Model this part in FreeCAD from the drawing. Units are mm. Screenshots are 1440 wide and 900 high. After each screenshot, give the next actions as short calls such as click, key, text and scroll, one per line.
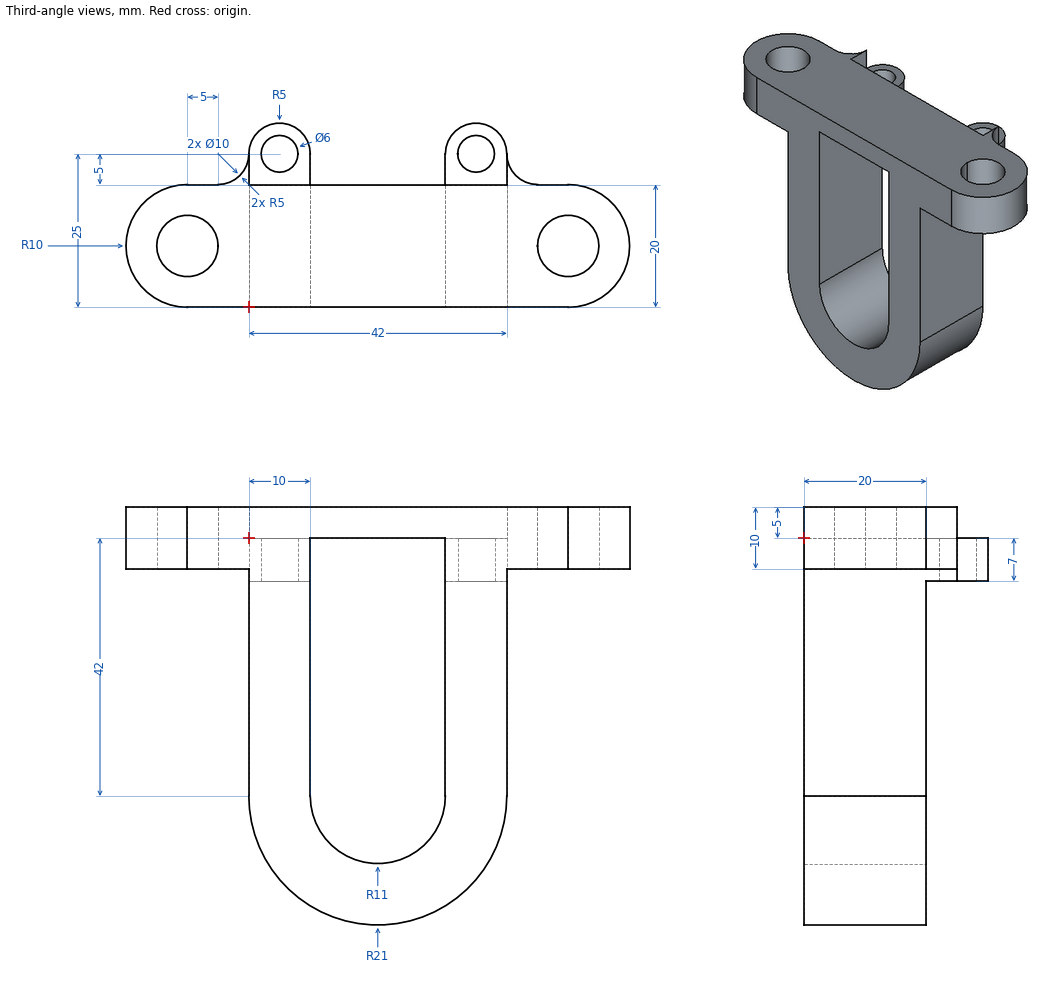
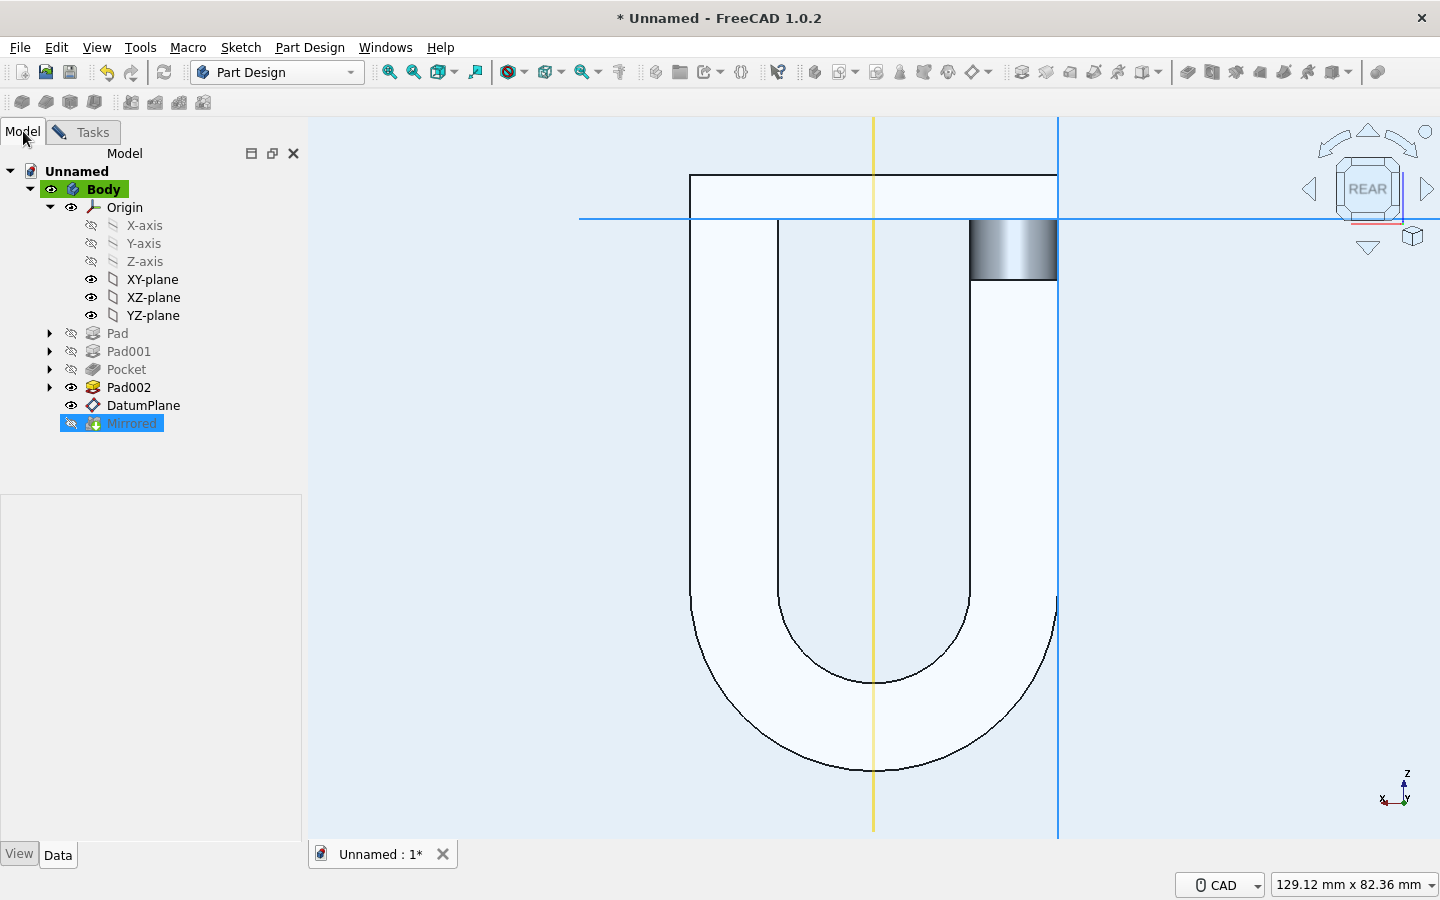
click(116, 405)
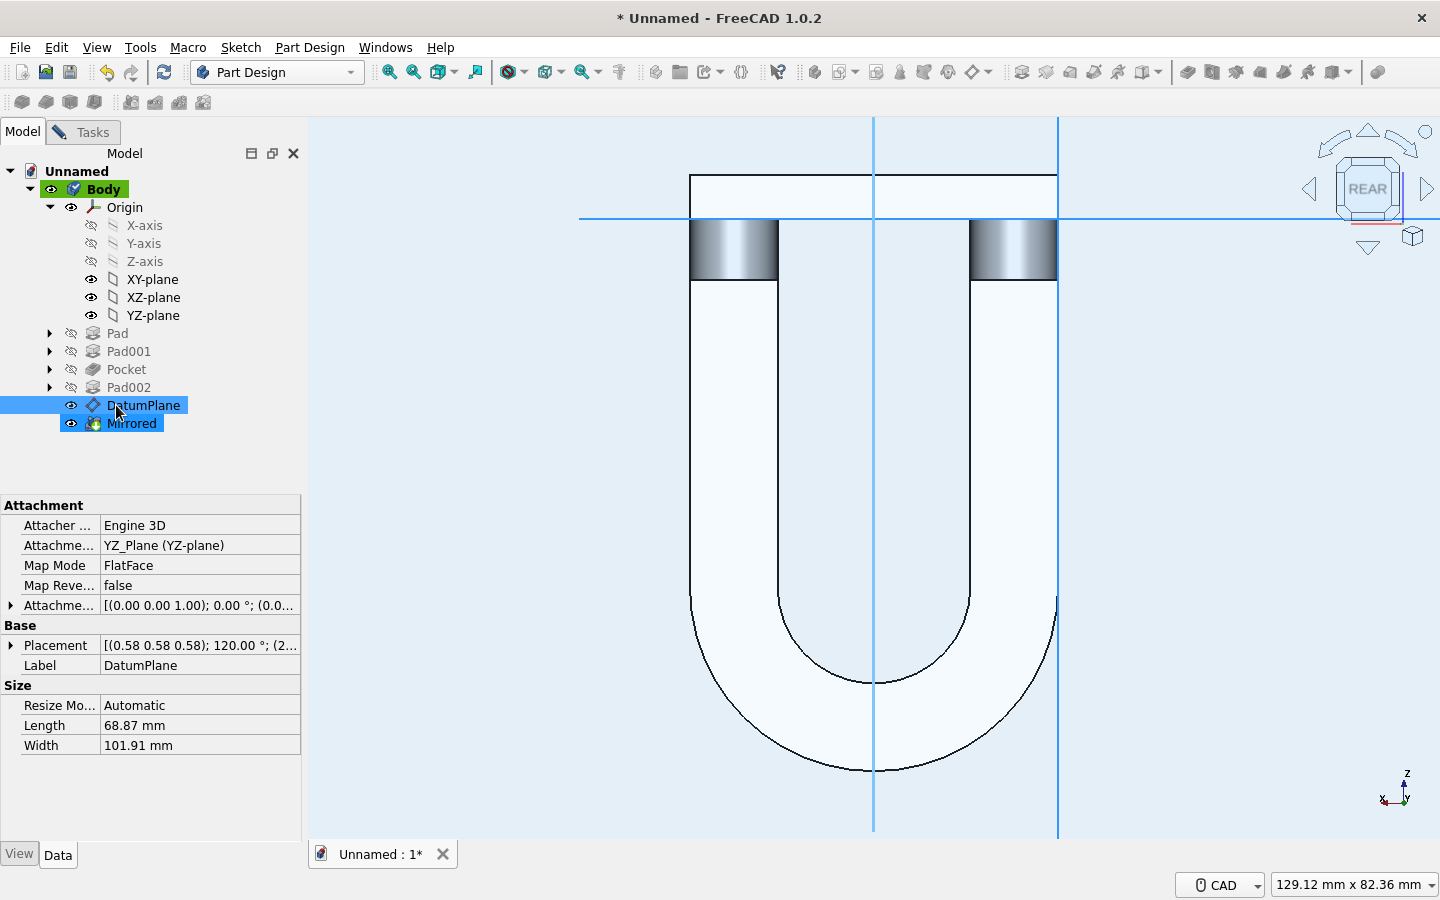
click(84, 131)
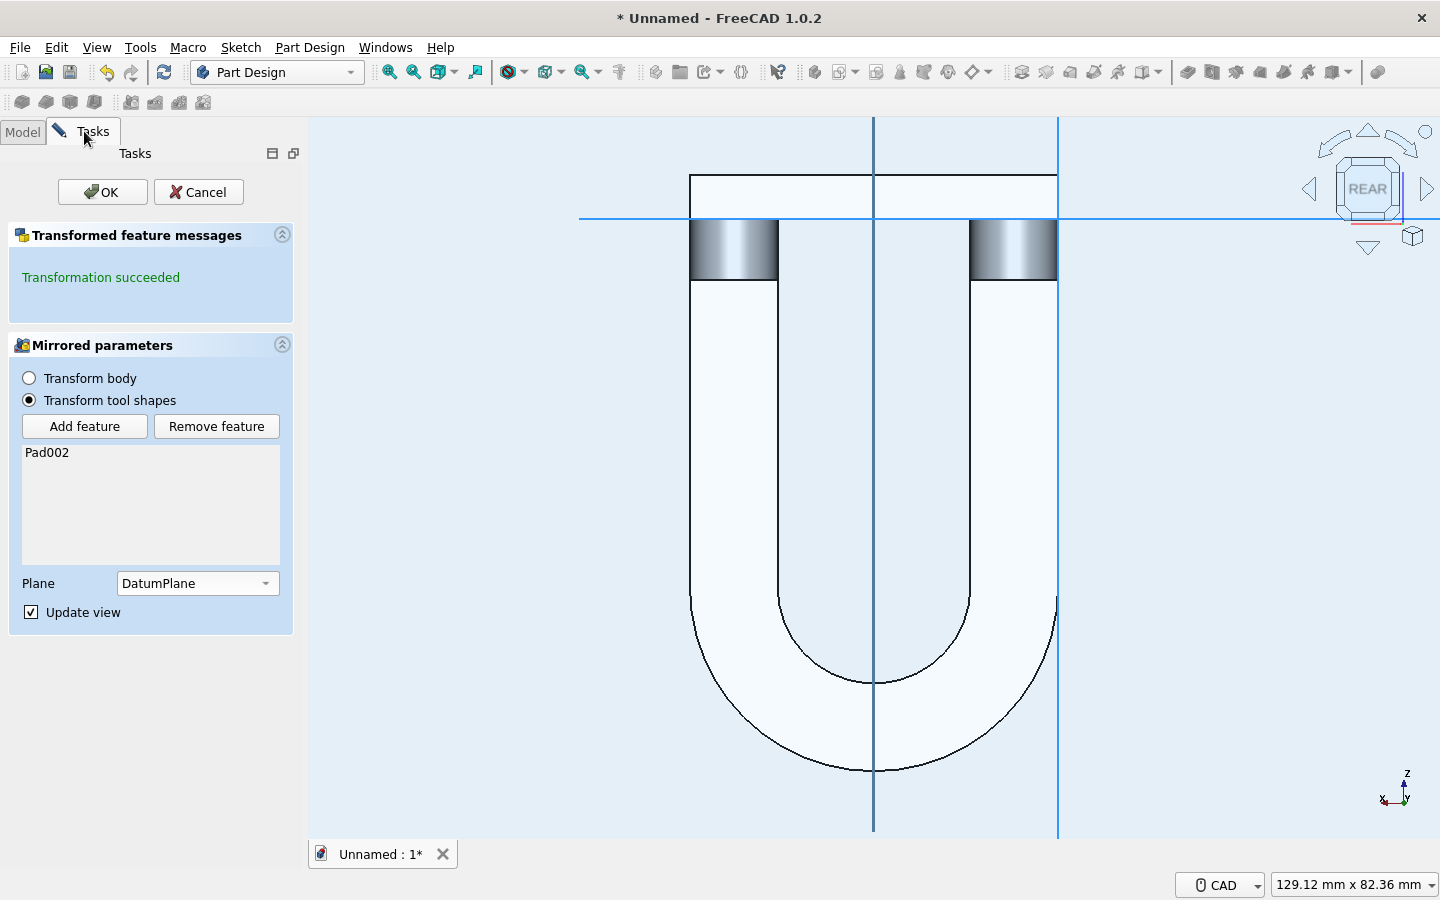
click(103, 192)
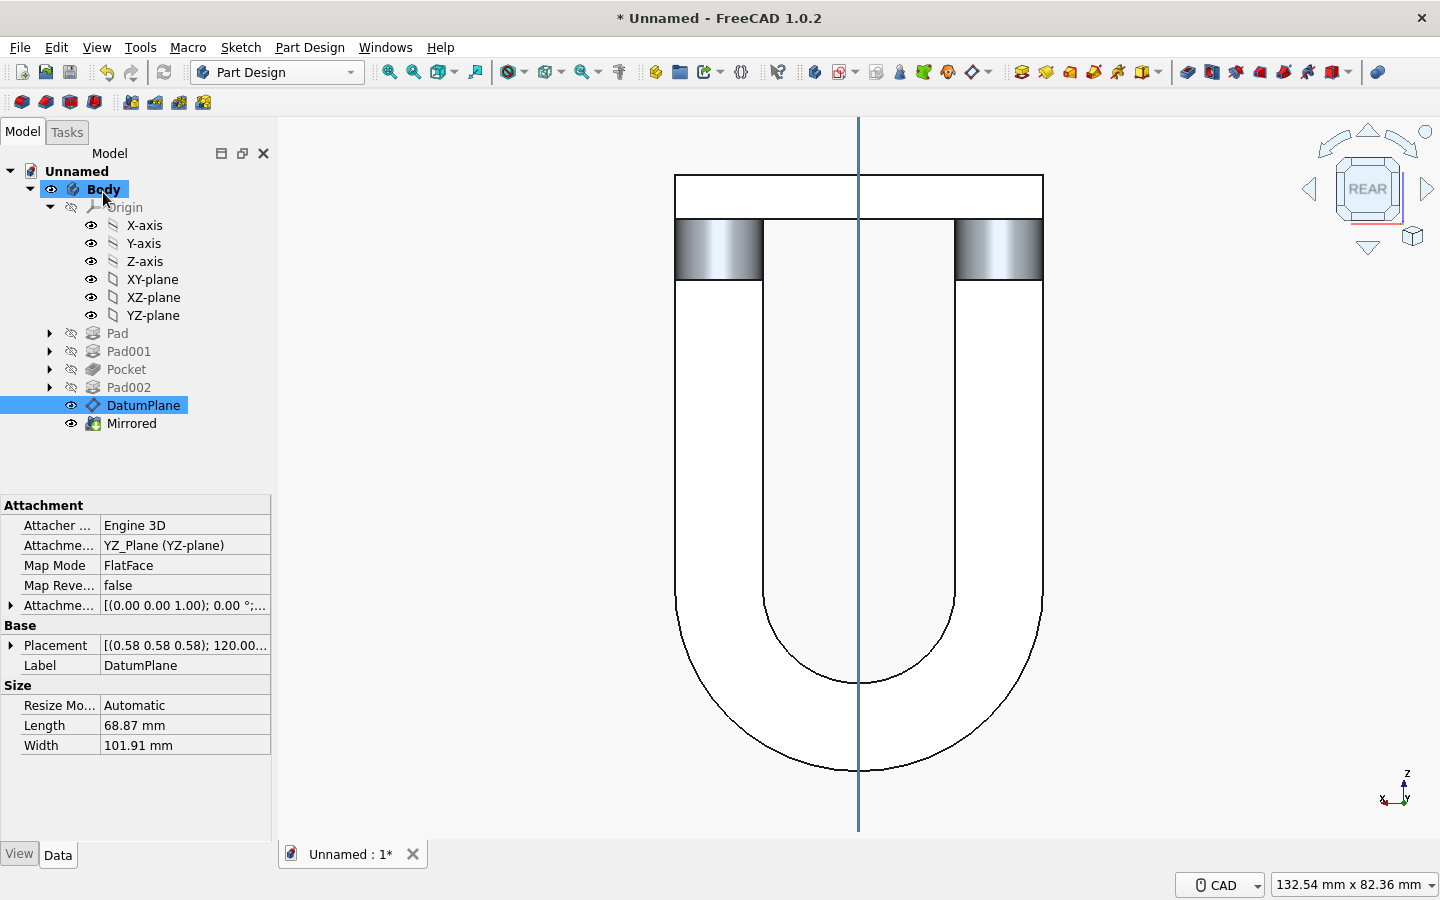
click(116, 405)
key(space)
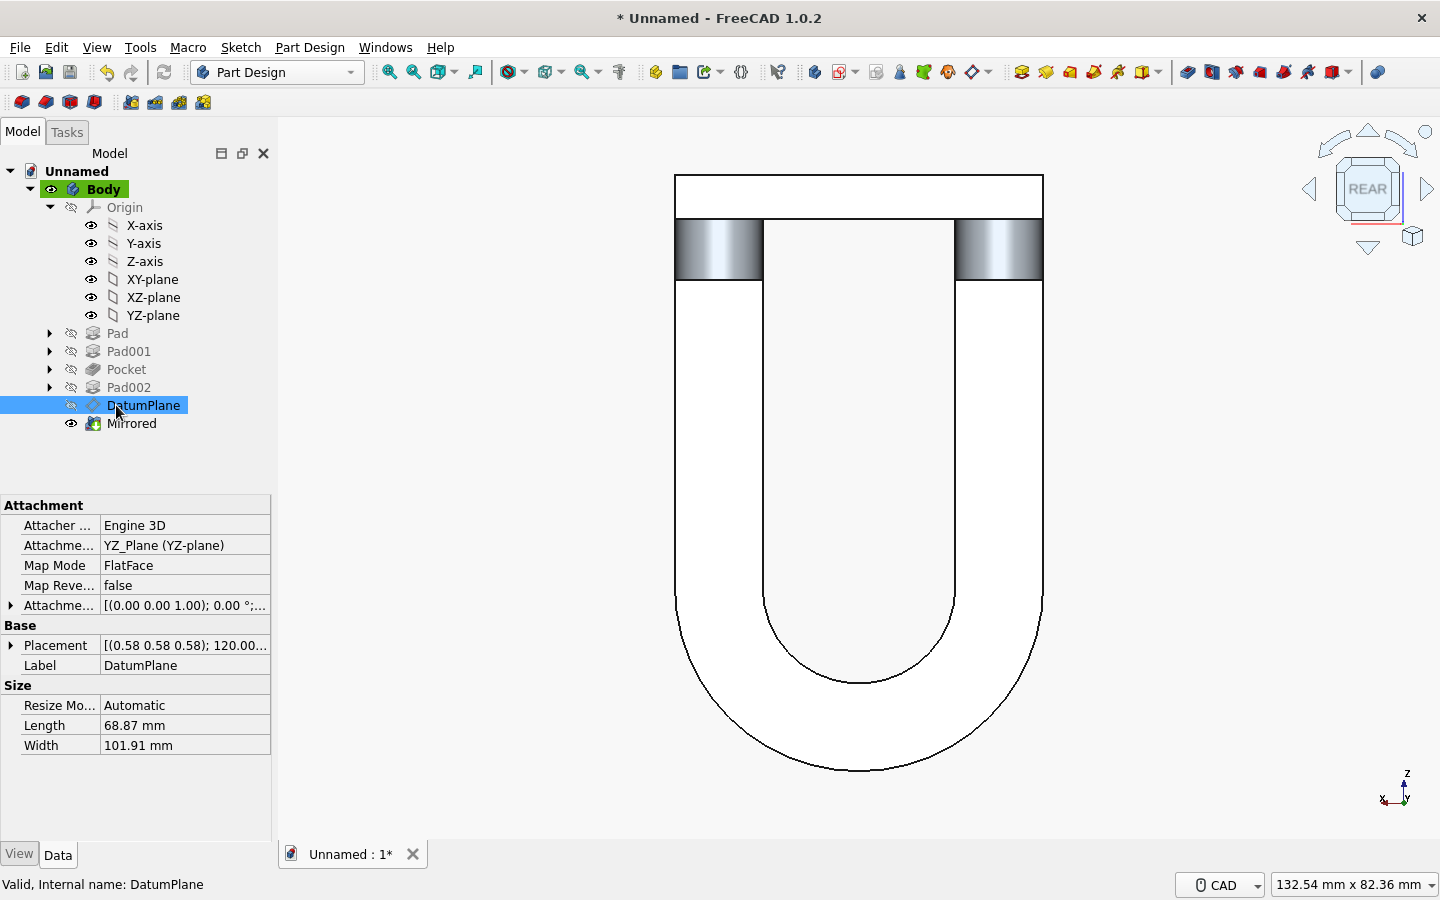
click(318, 799)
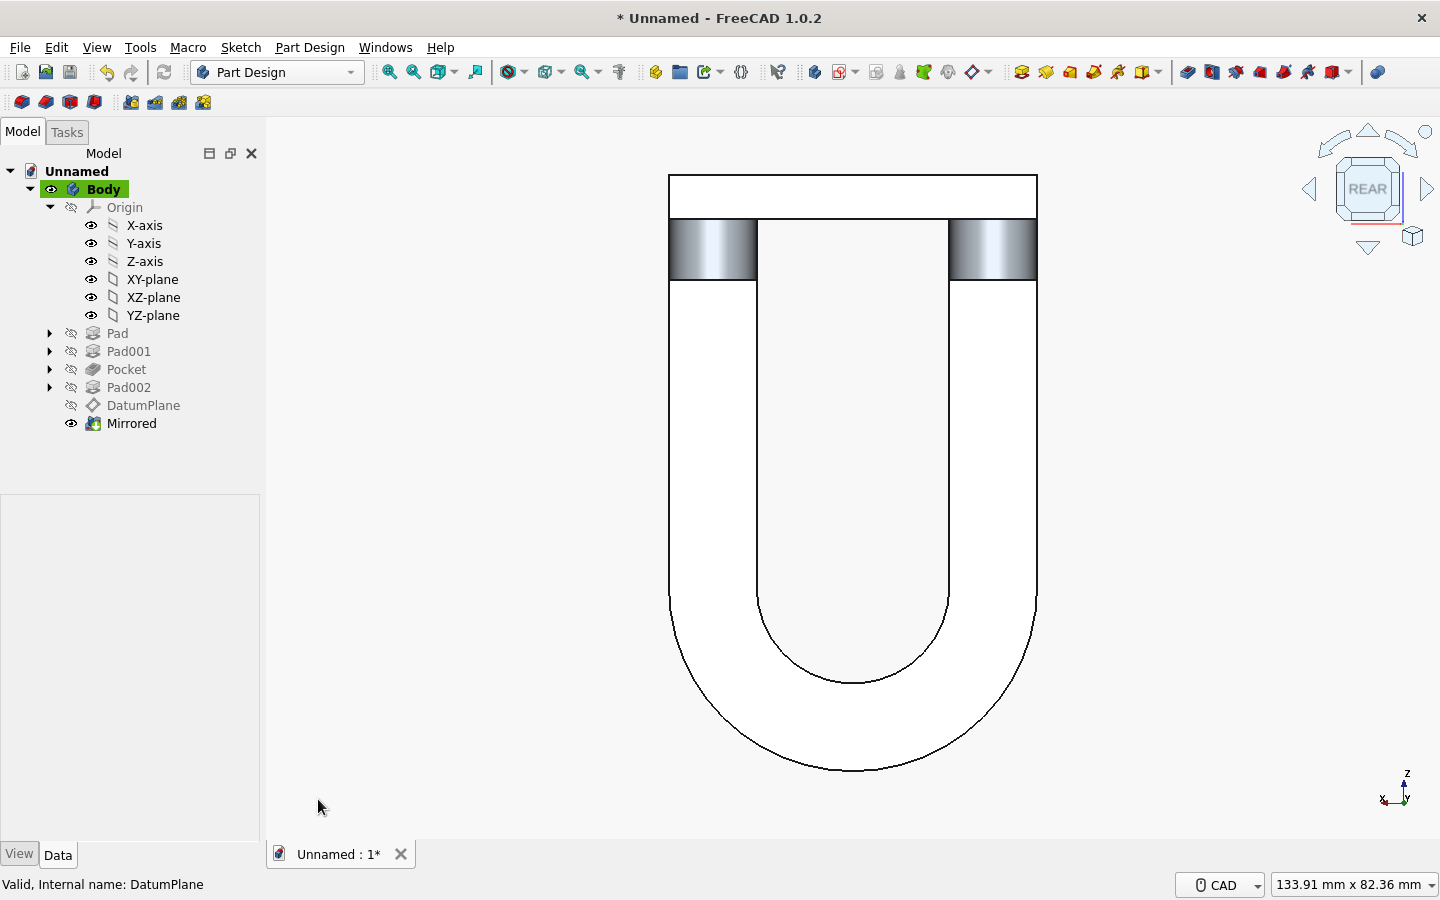
click(840, 72)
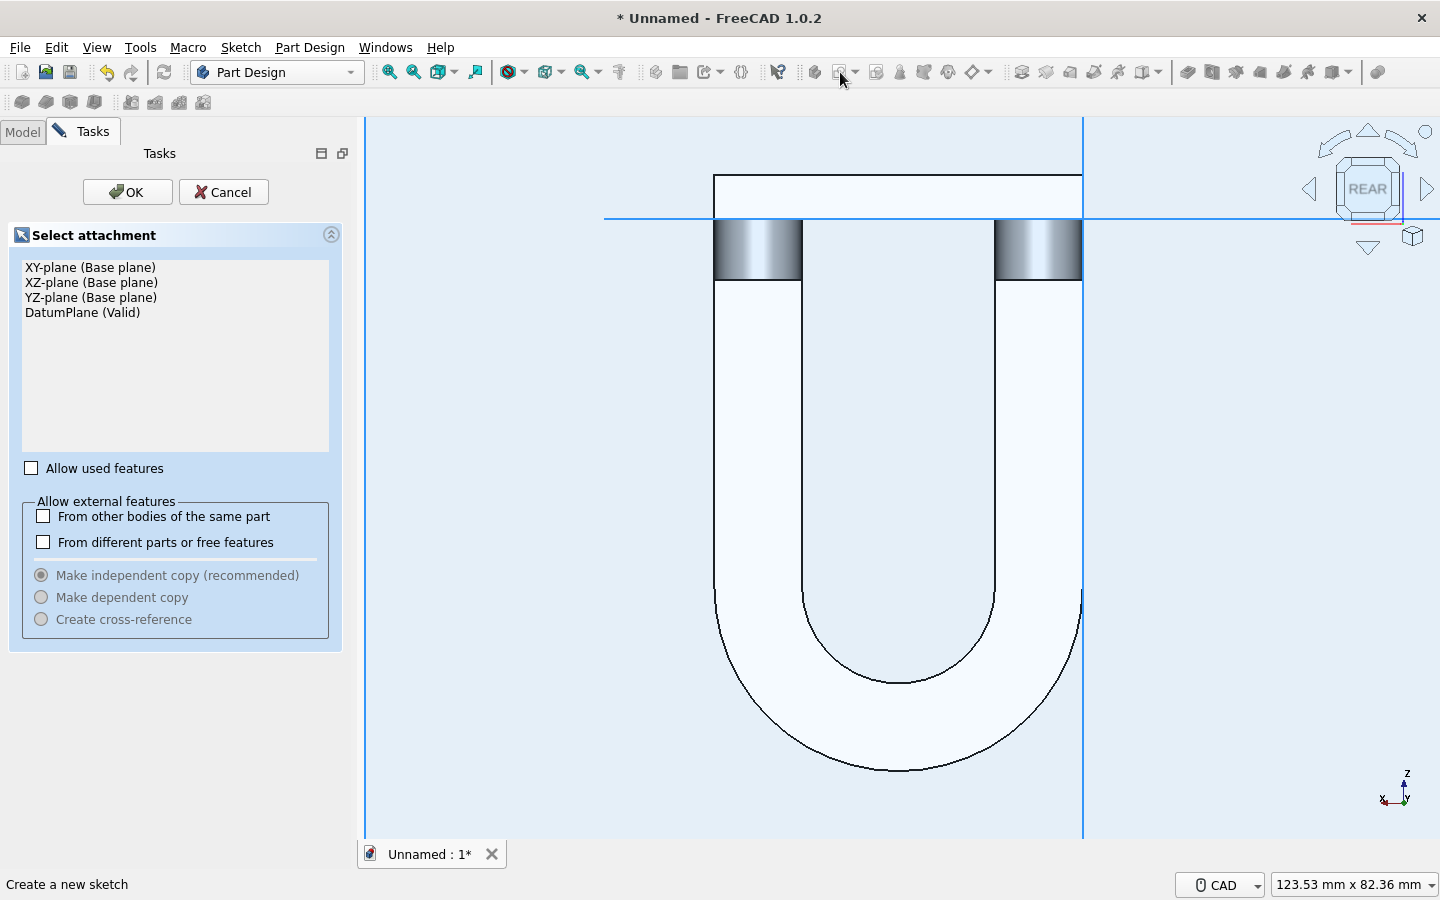
click(82, 268)